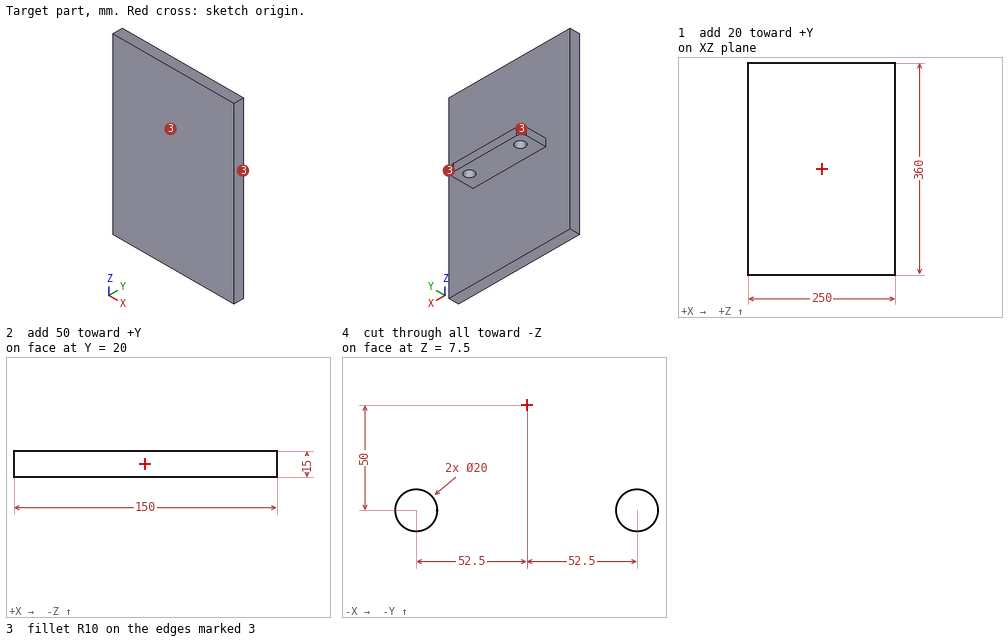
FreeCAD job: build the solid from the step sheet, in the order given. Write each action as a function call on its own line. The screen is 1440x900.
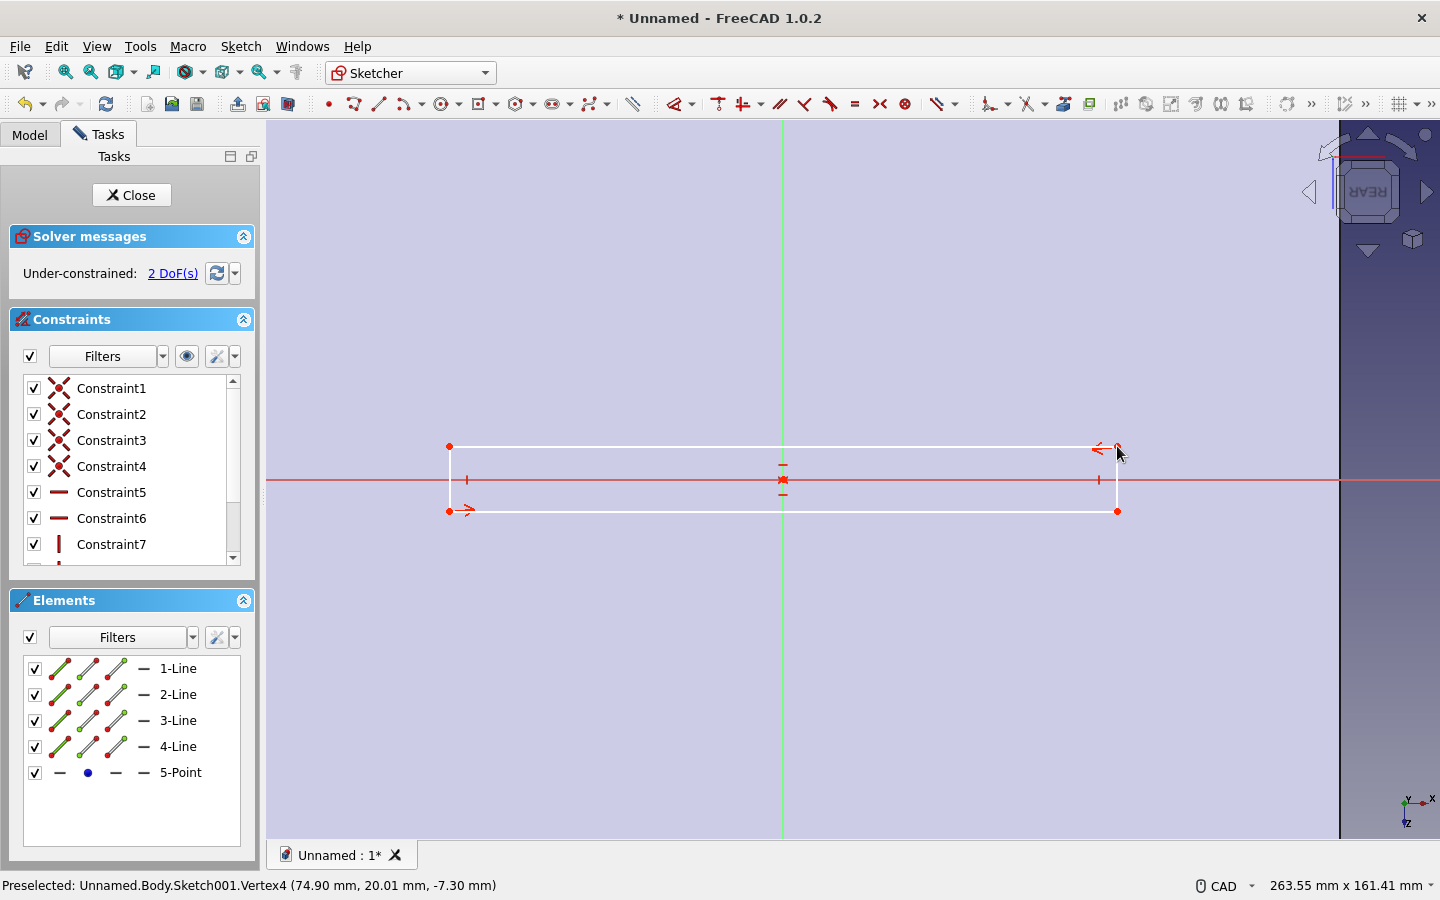
key(d)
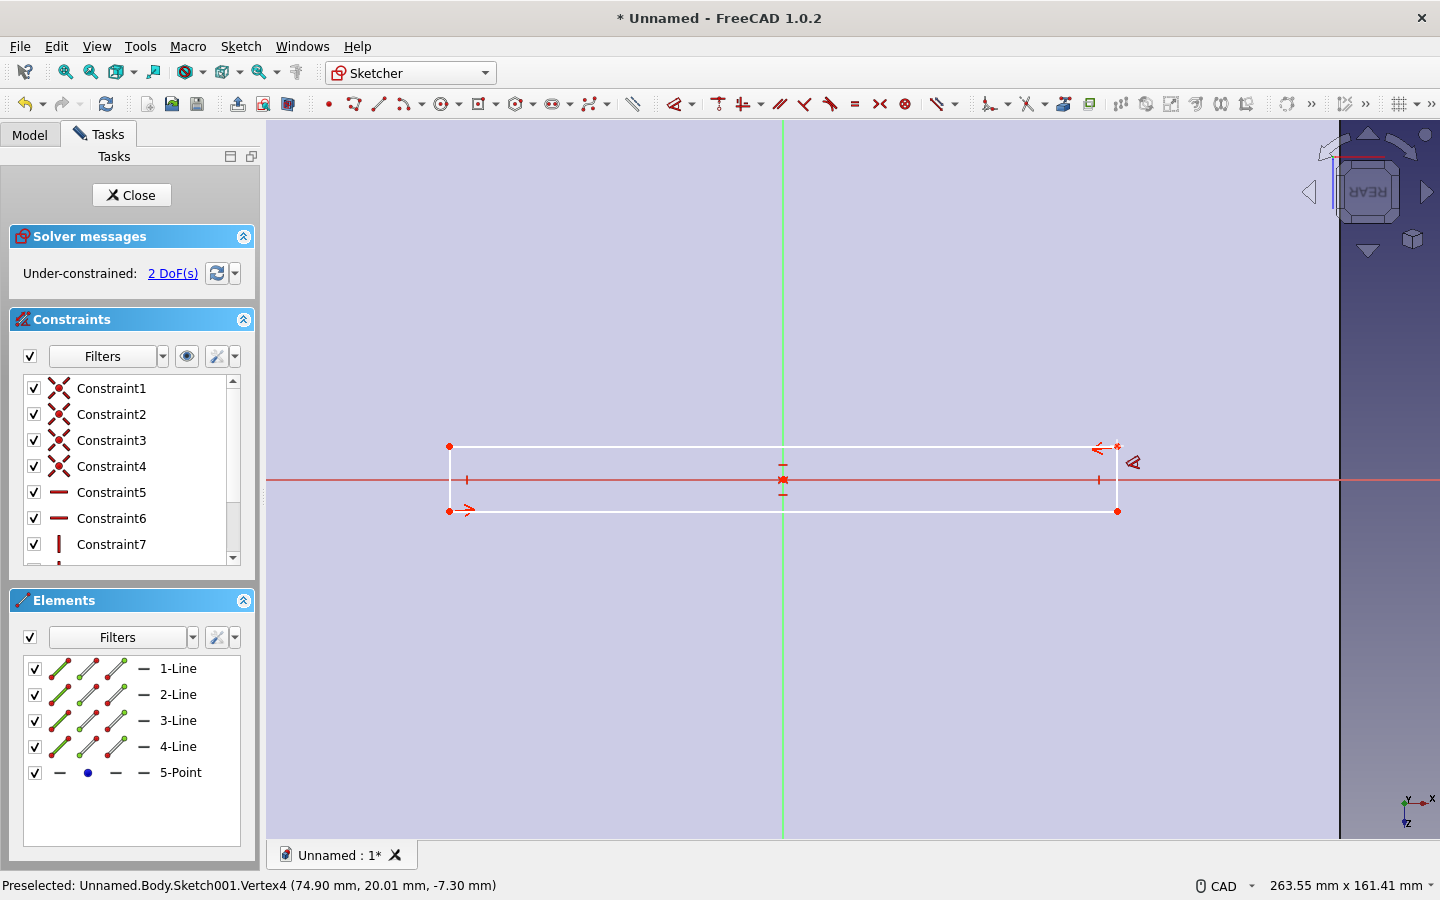
click(1117, 492)
click(1151, 465)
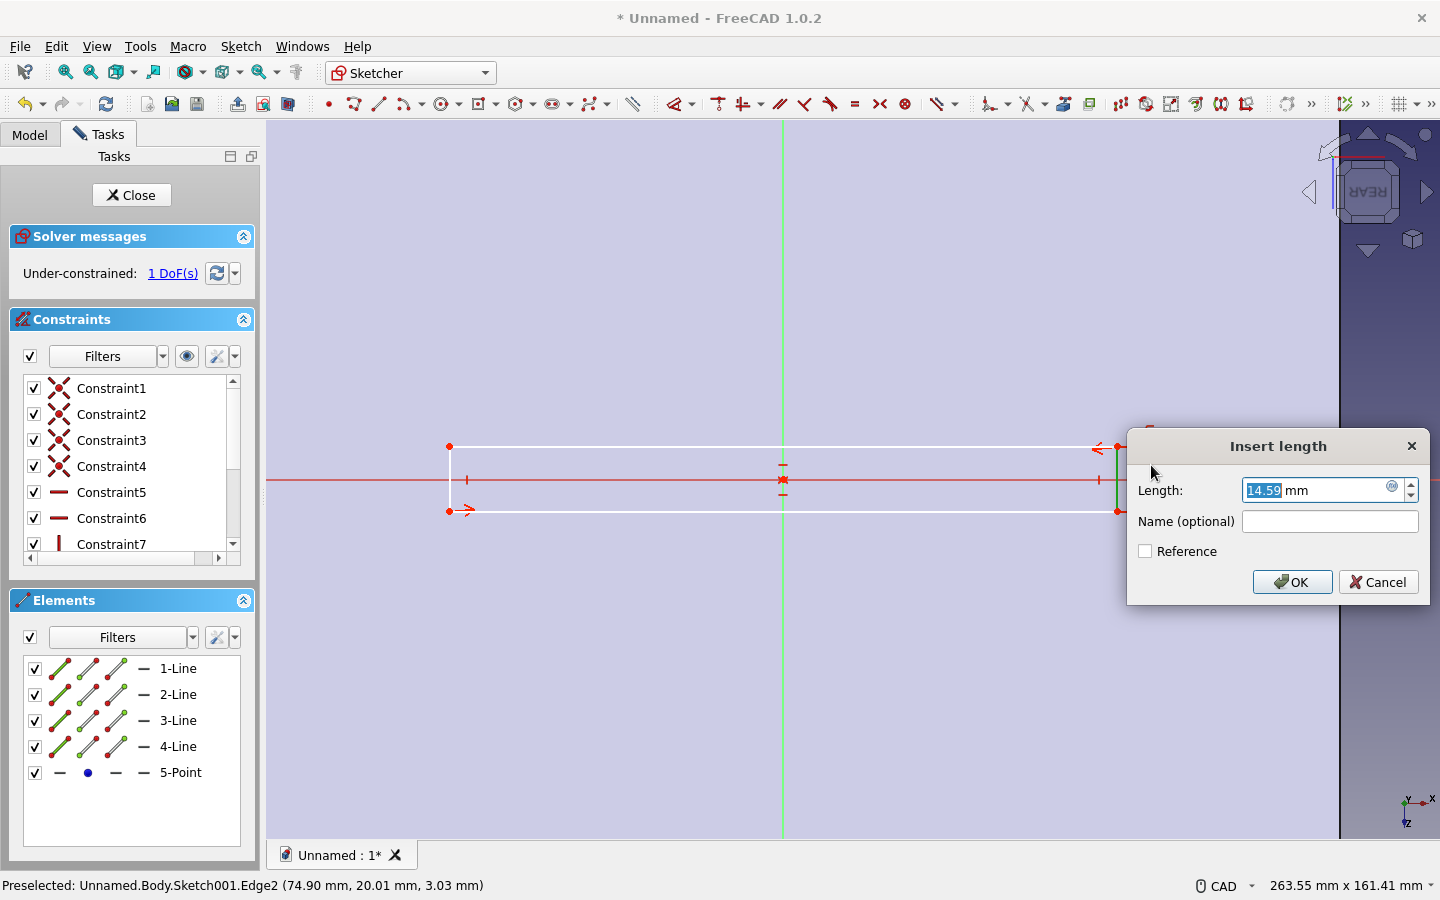
text(15)
key(Return)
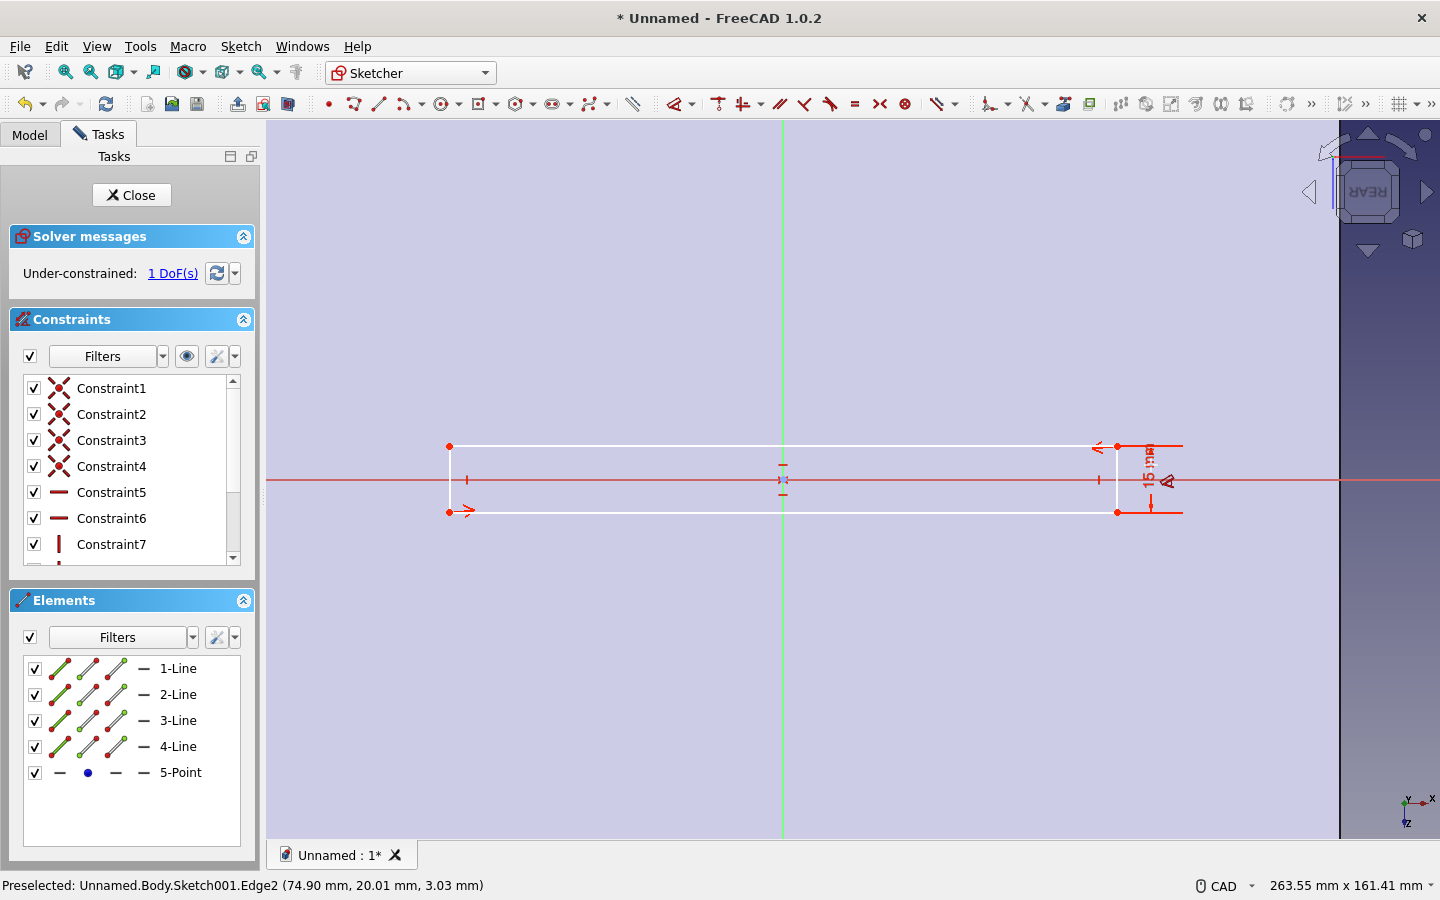
click(650, 513)
click(630, 547)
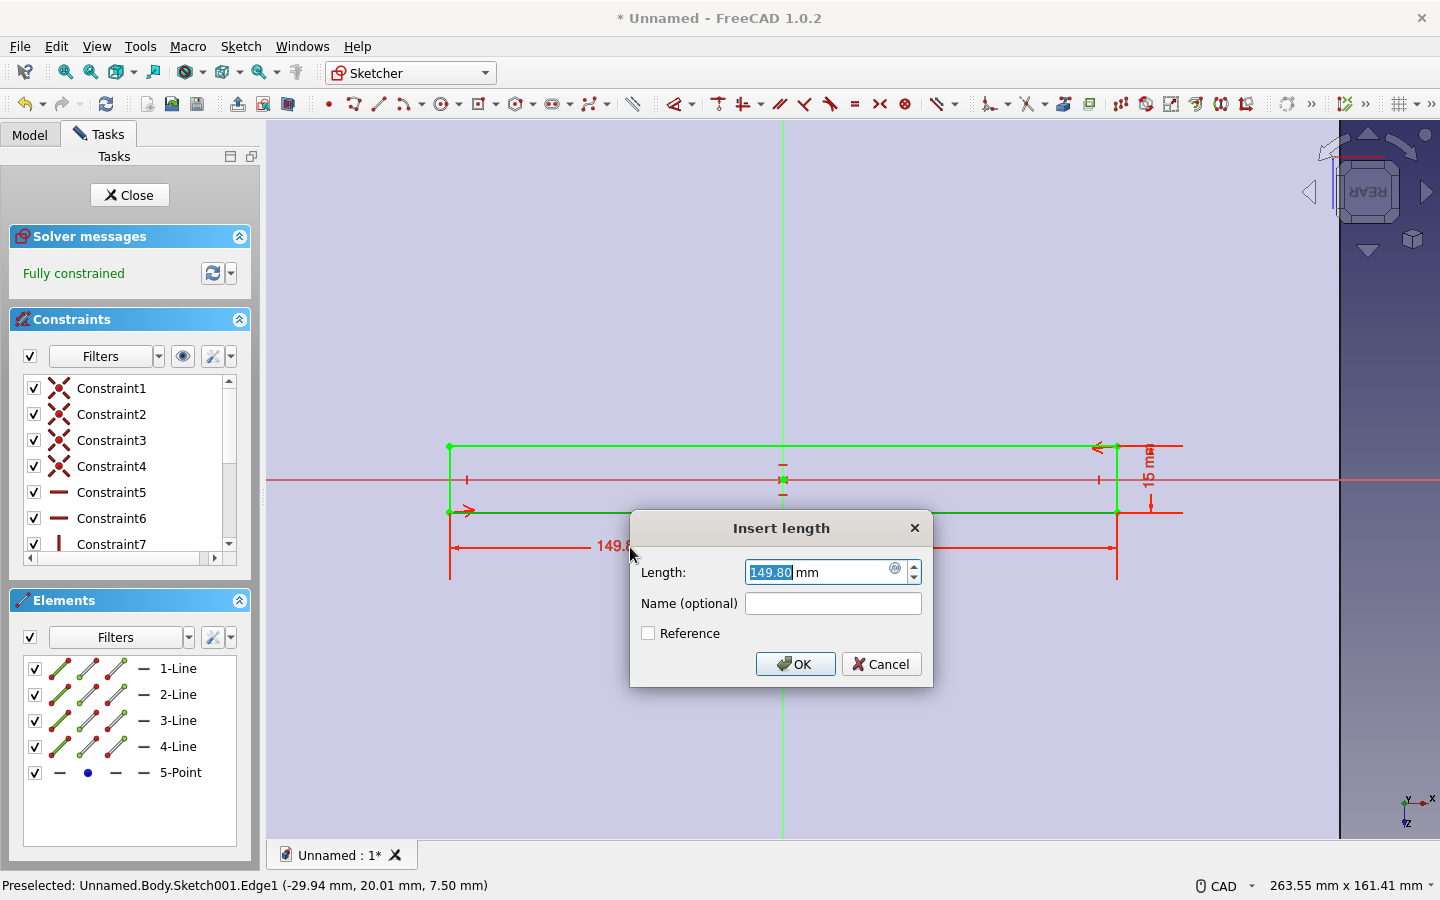
text(150)
key(Return)
key(Escape)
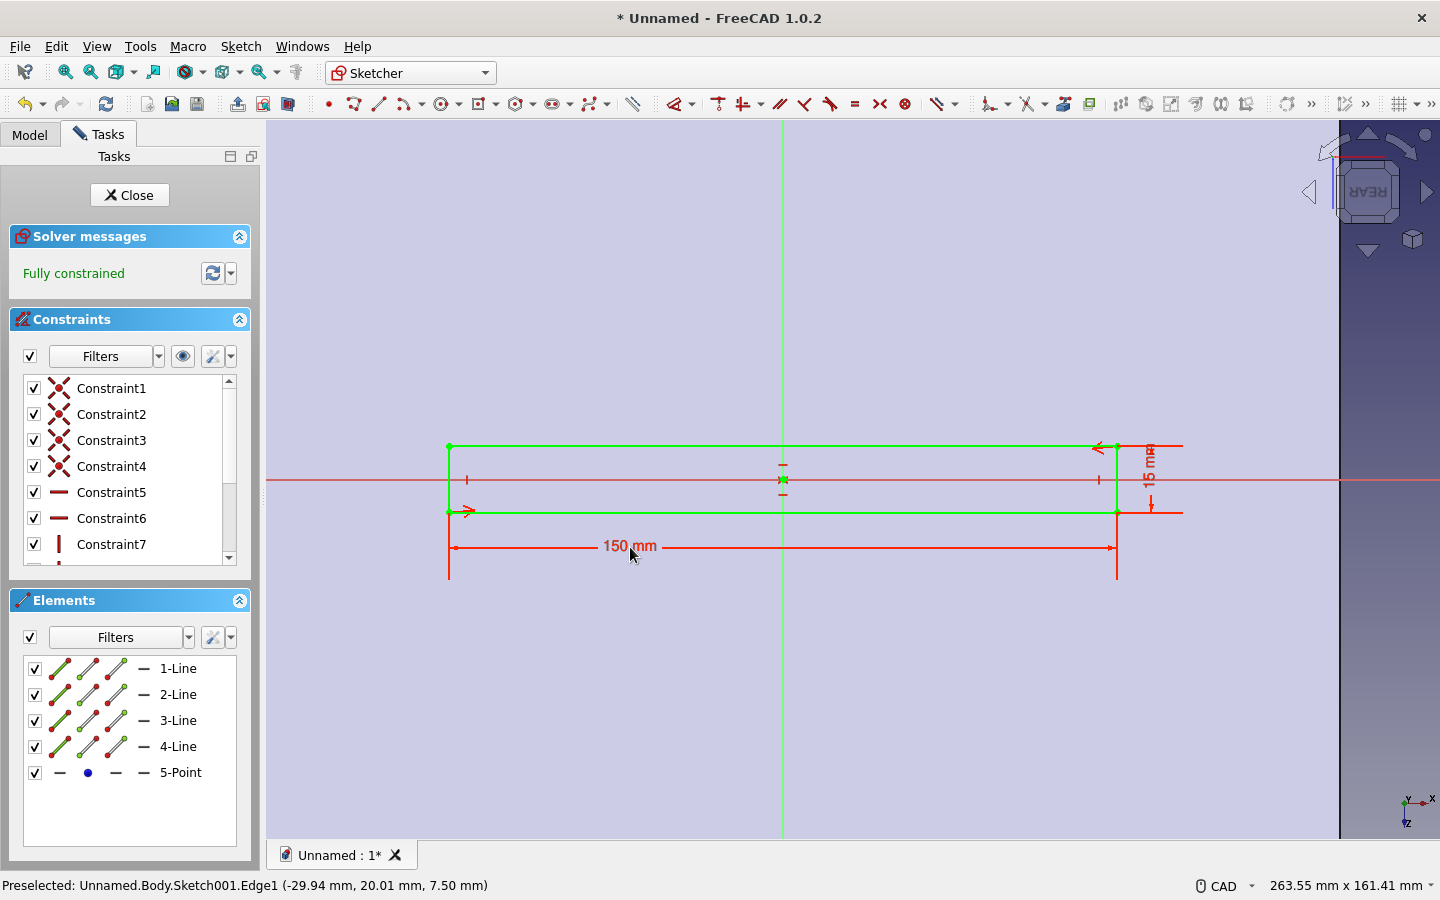
click(130, 195)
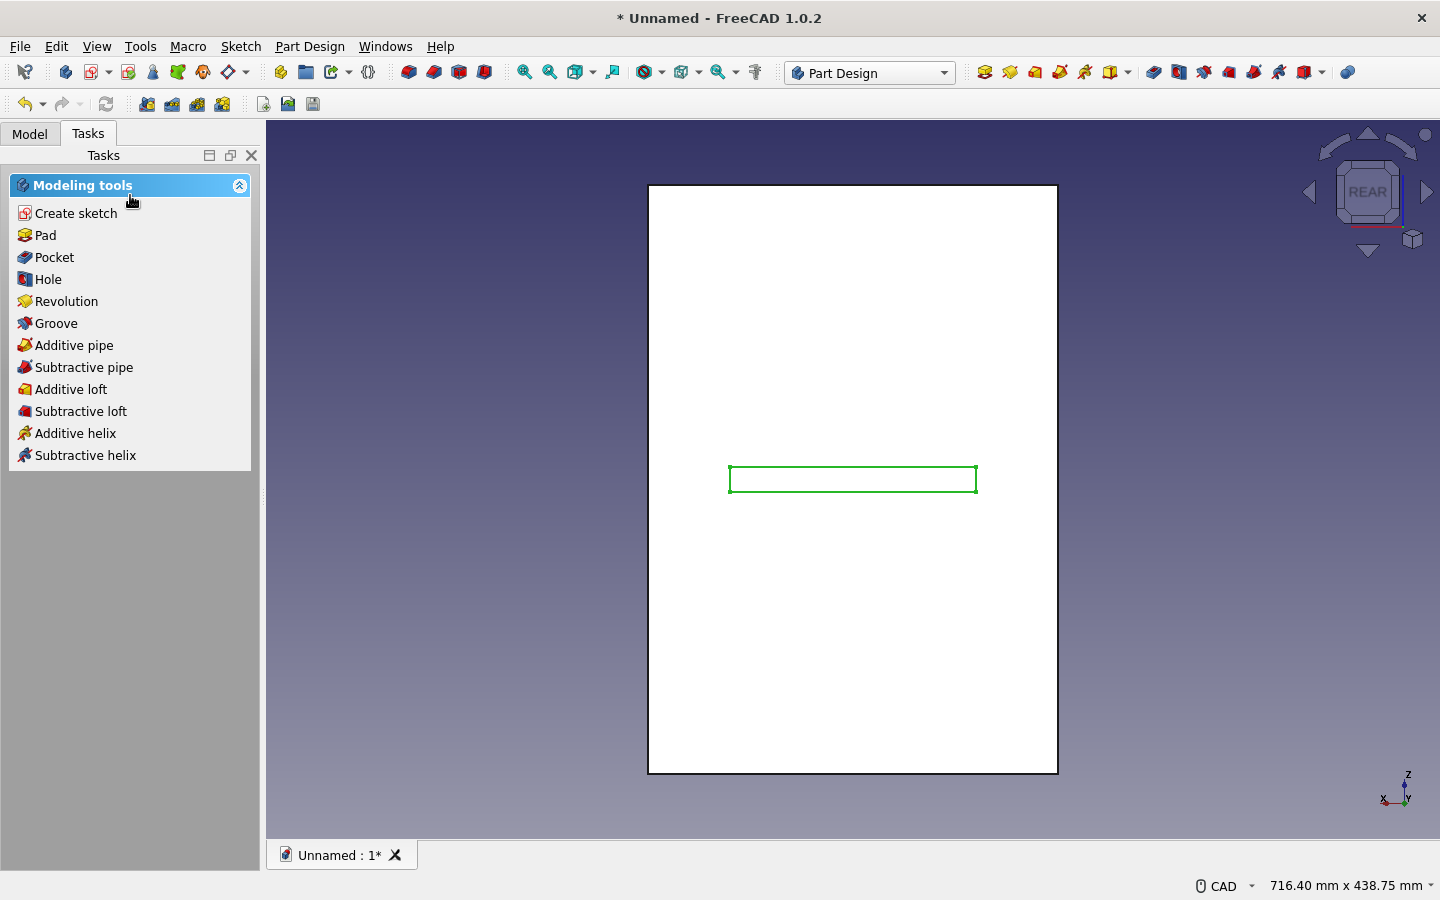
click(985, 72)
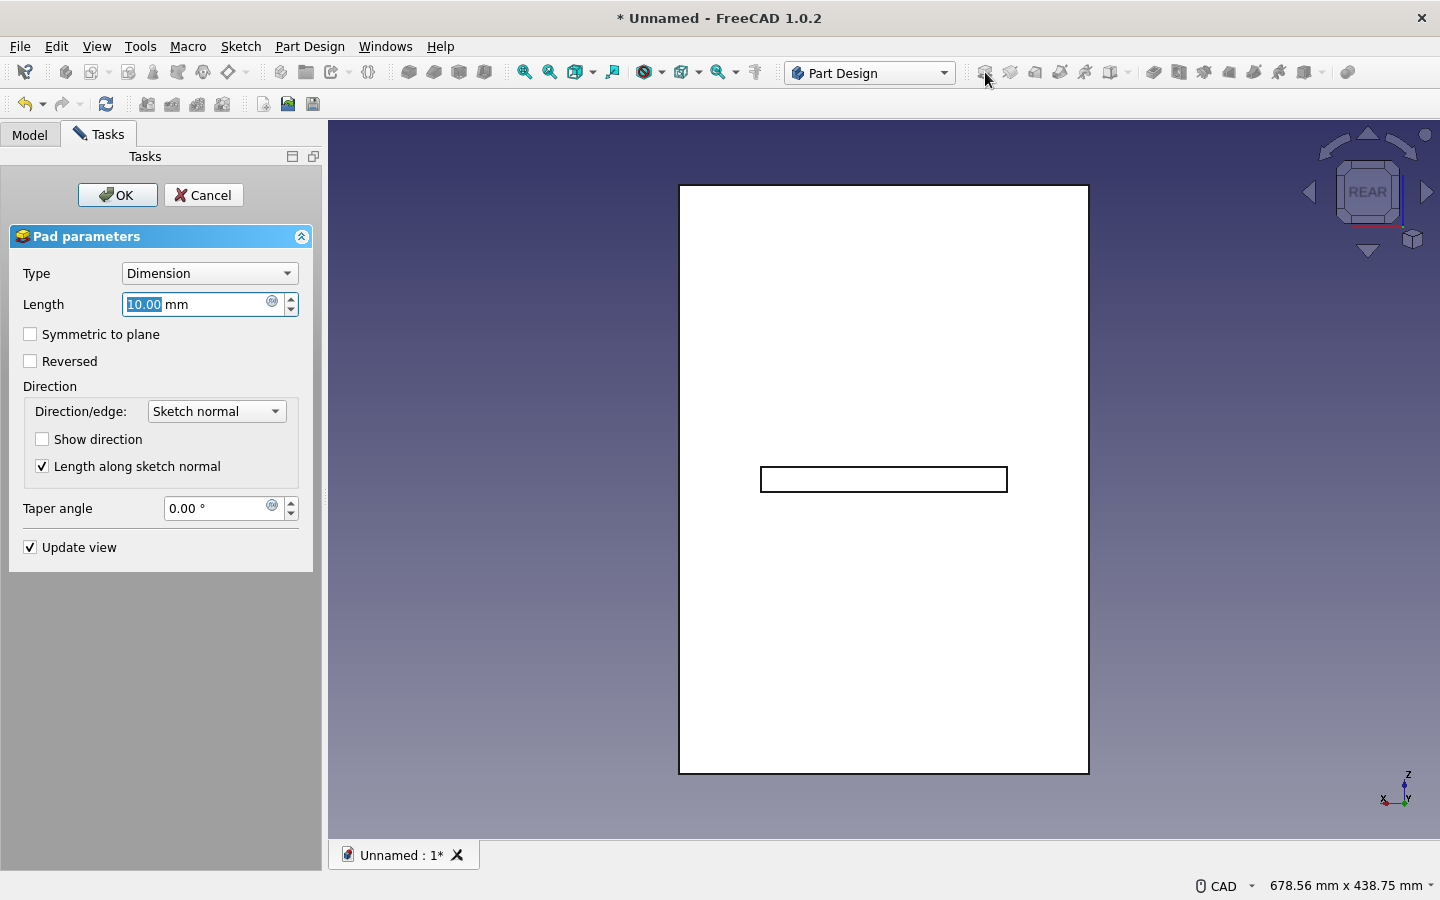
text(50)
key(Tab)